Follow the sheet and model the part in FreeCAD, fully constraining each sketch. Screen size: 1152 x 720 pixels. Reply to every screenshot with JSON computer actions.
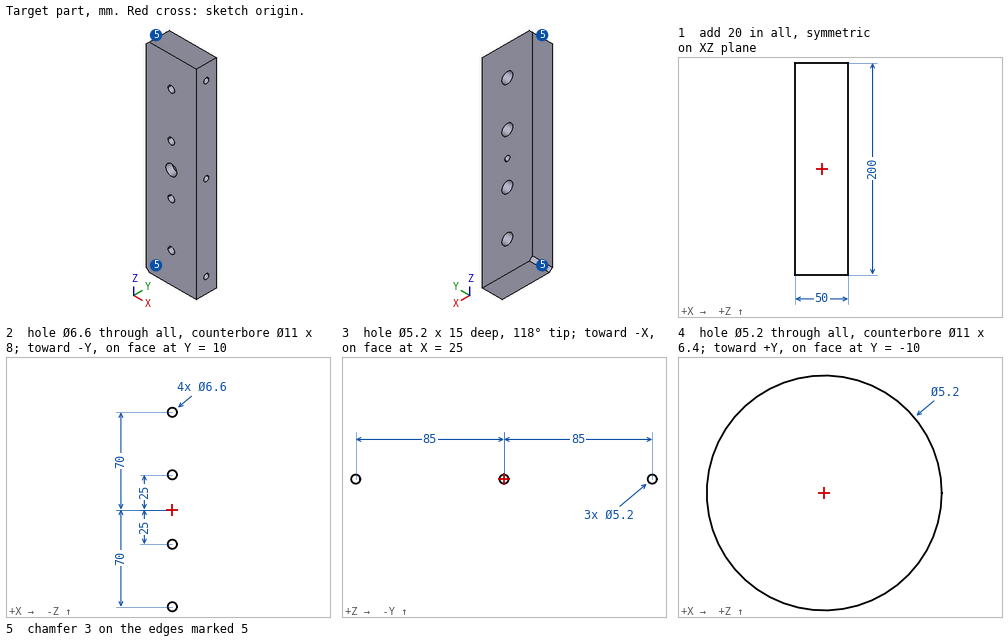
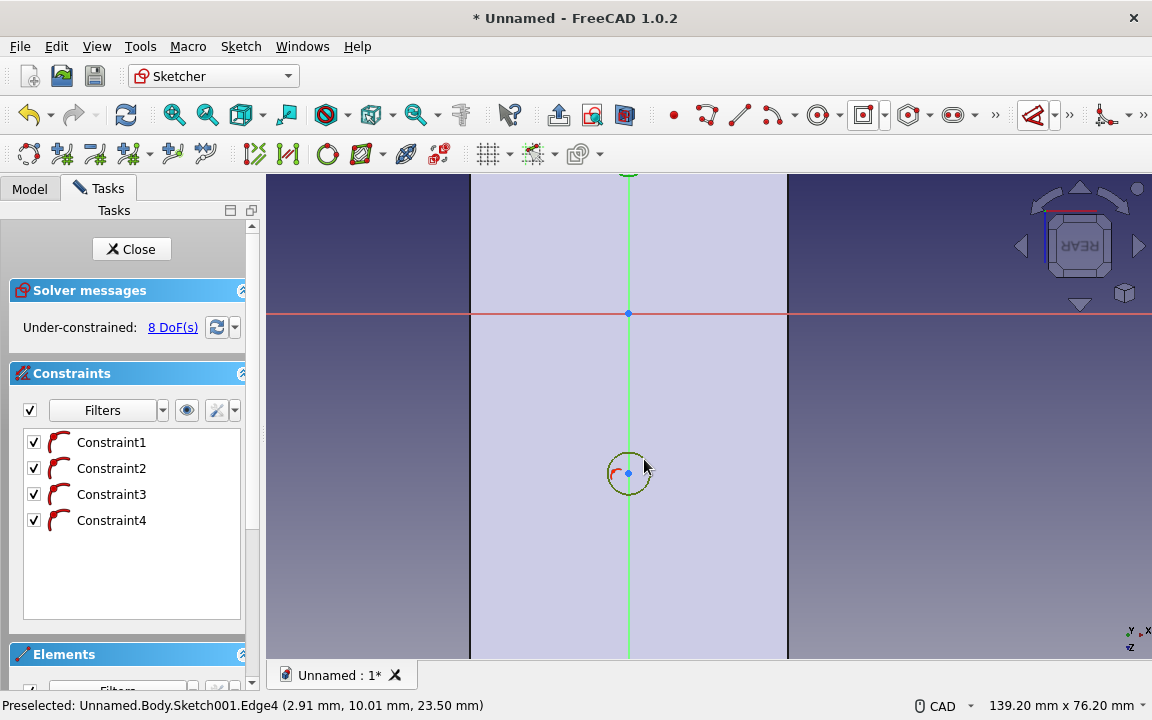
{"action": "key", "text": "e"}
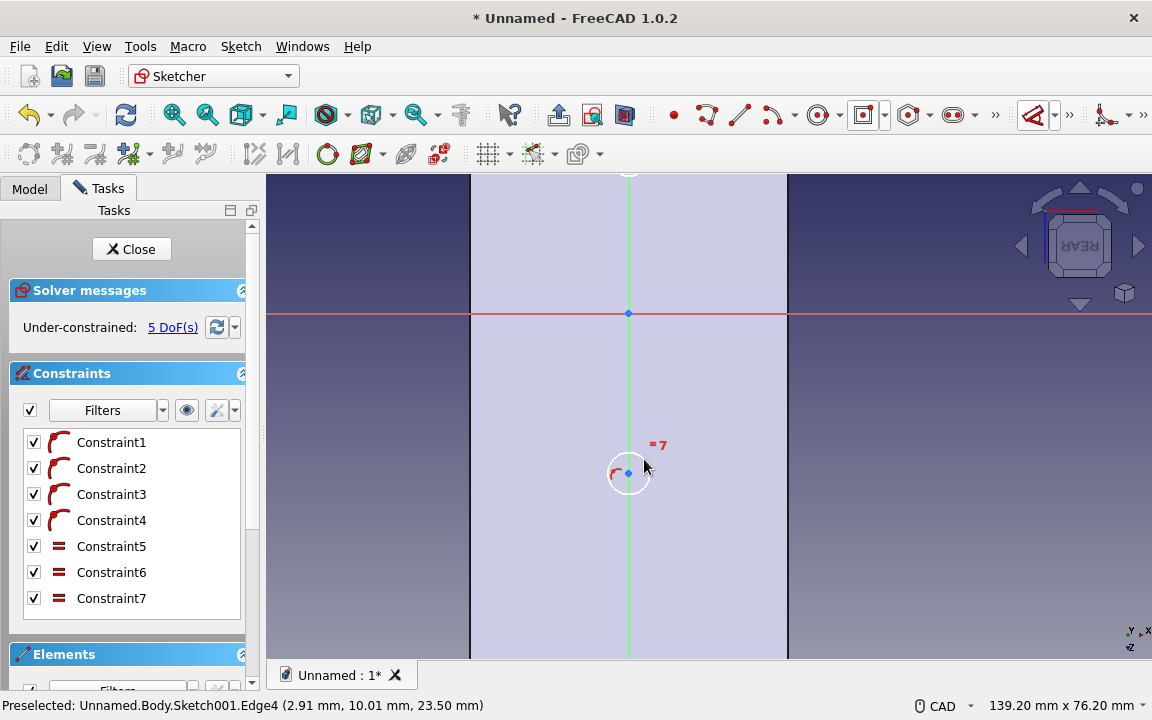
{"action": "scroll", "coordinate": [645, 461], "scroll_direction": "down", "scroll_amount": 6}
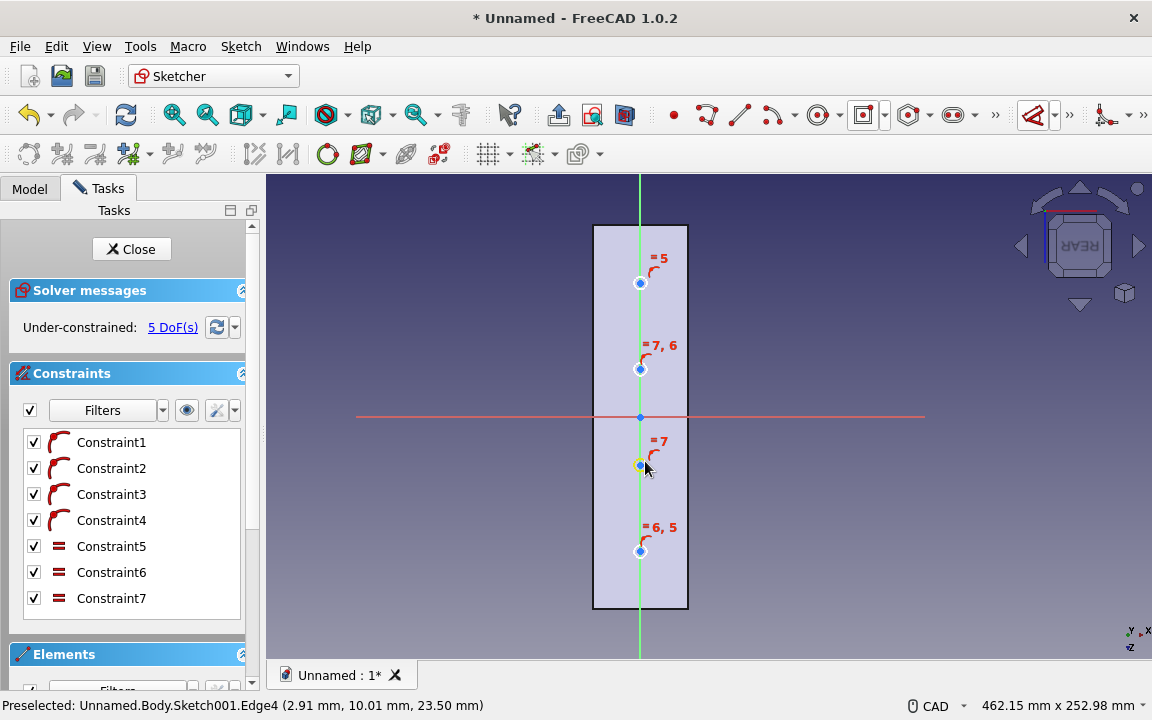
{"action": "scroll", "coordinate": [645, 279], "scroll_direction": "up", "scroll_amount": 6}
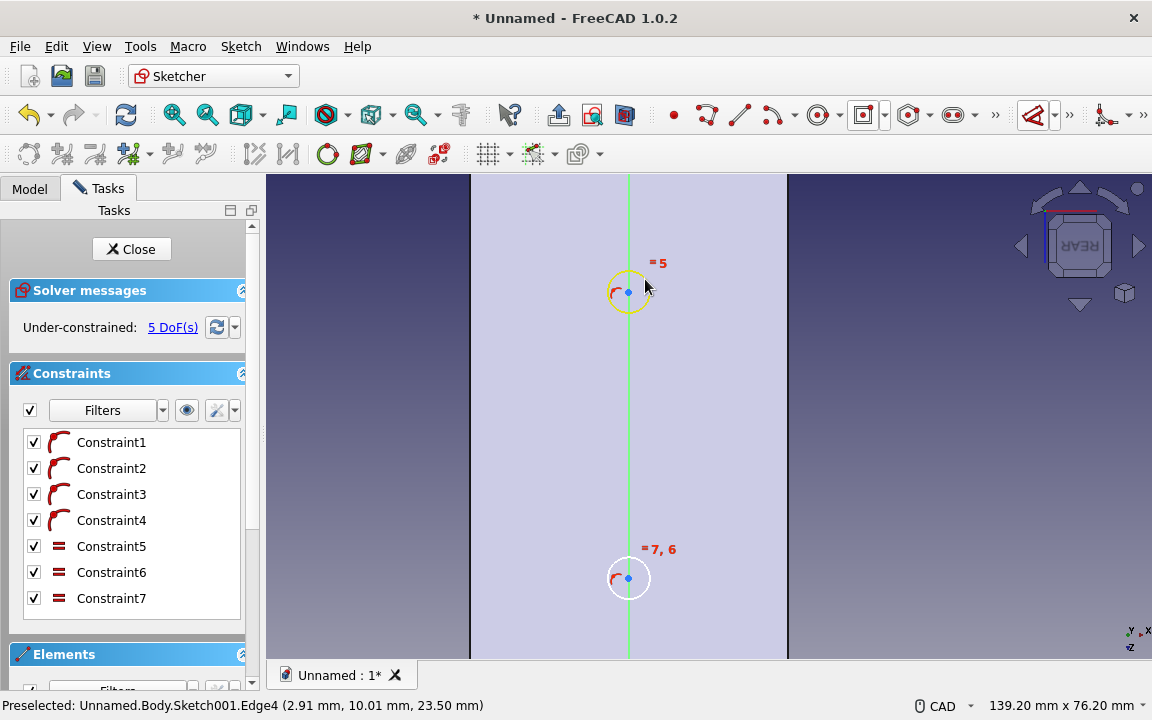
{"action": "left_click", "coordinate": [644, 277]}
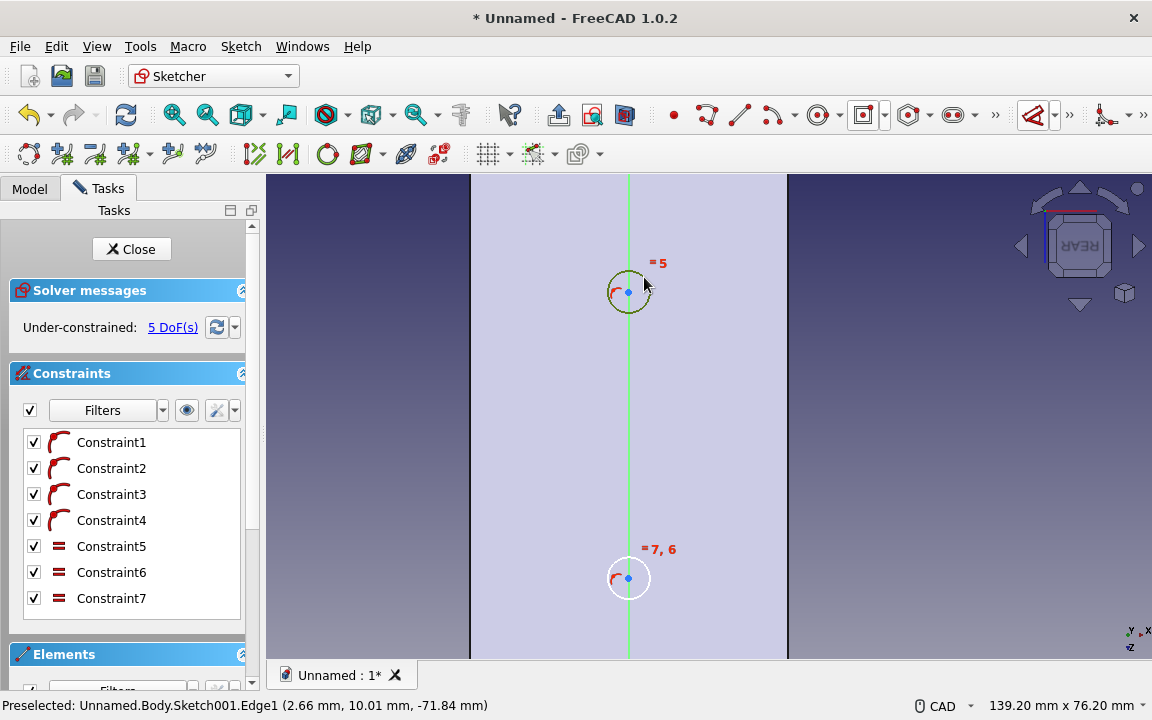
{"action": "left_click", "coordinate": [1054, 116]}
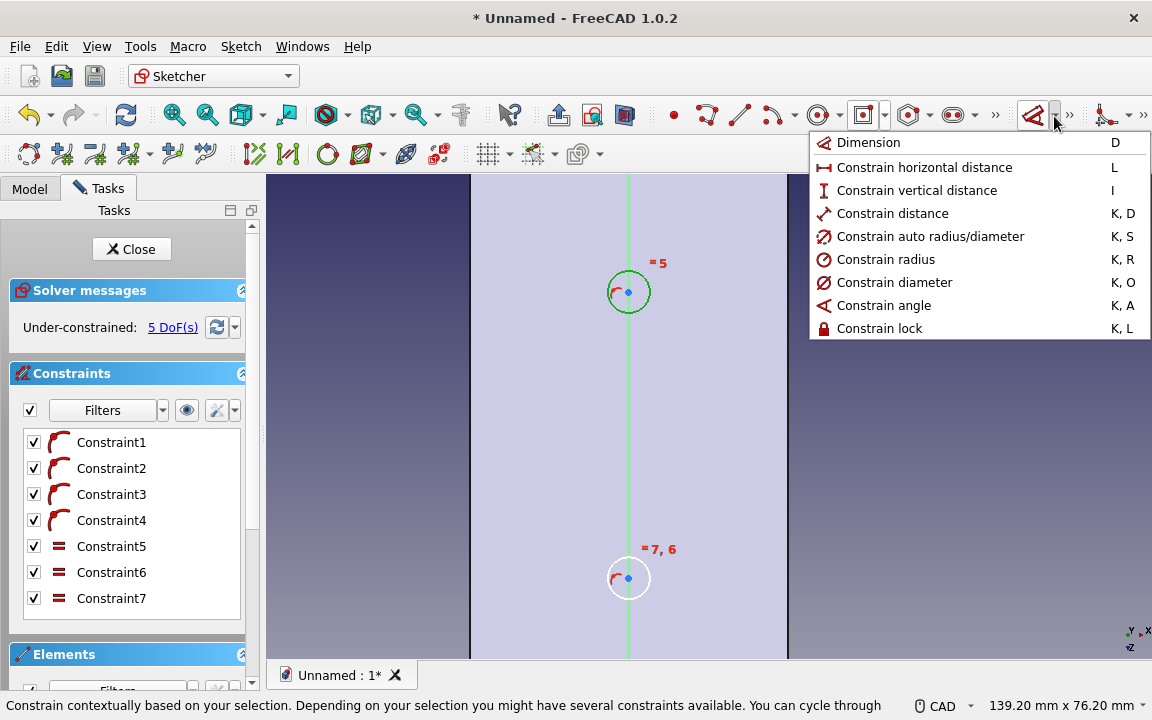
{"action": "left_click", "coordinate": [980, 282]}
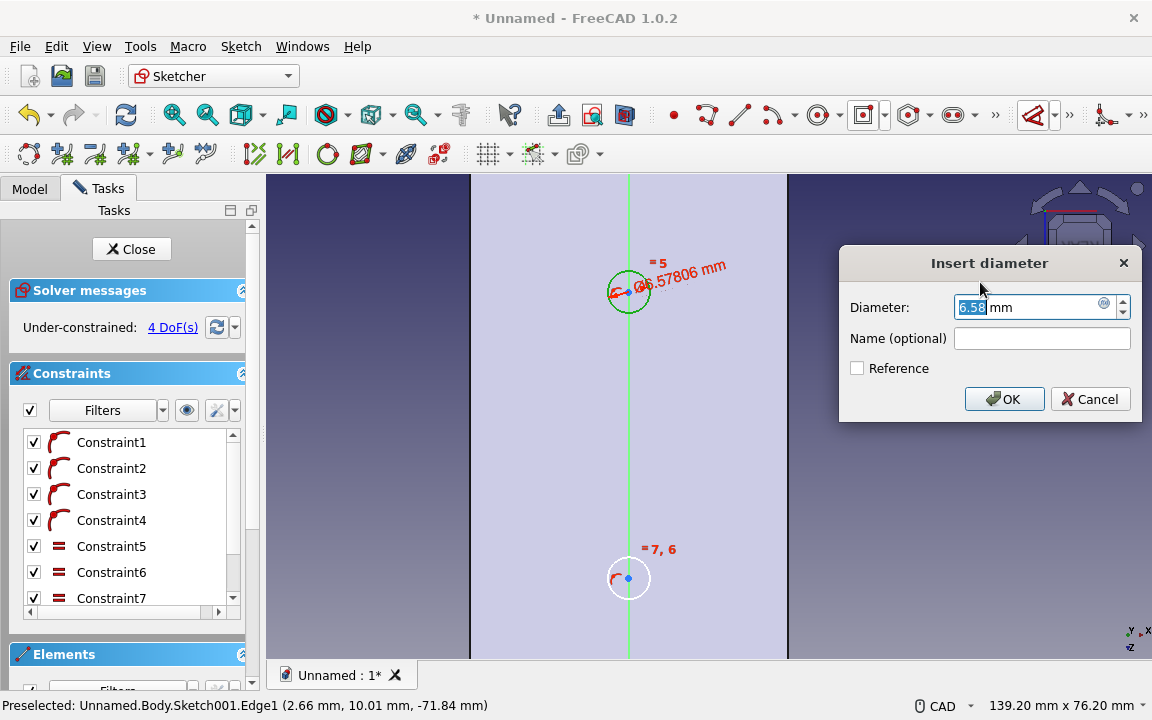
{"action": "type", "text": "6.6"}
{"action": "key", "text": "Return"}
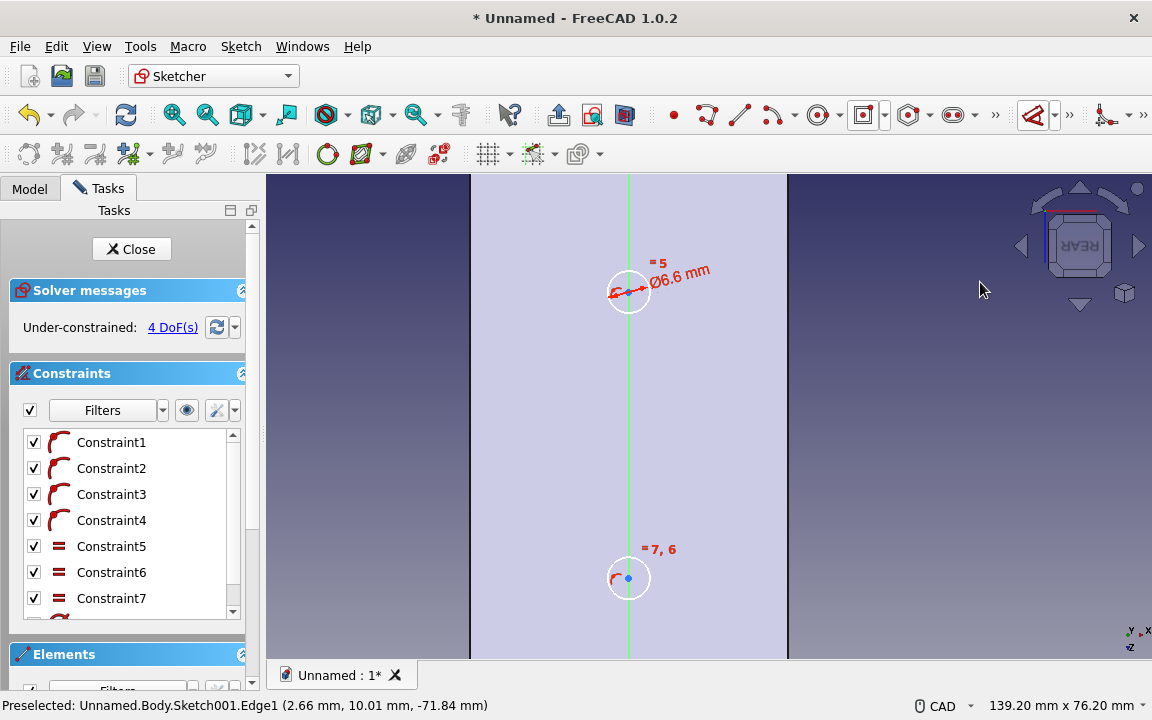
{"action": "left_click", "coordinate": [629, 292]}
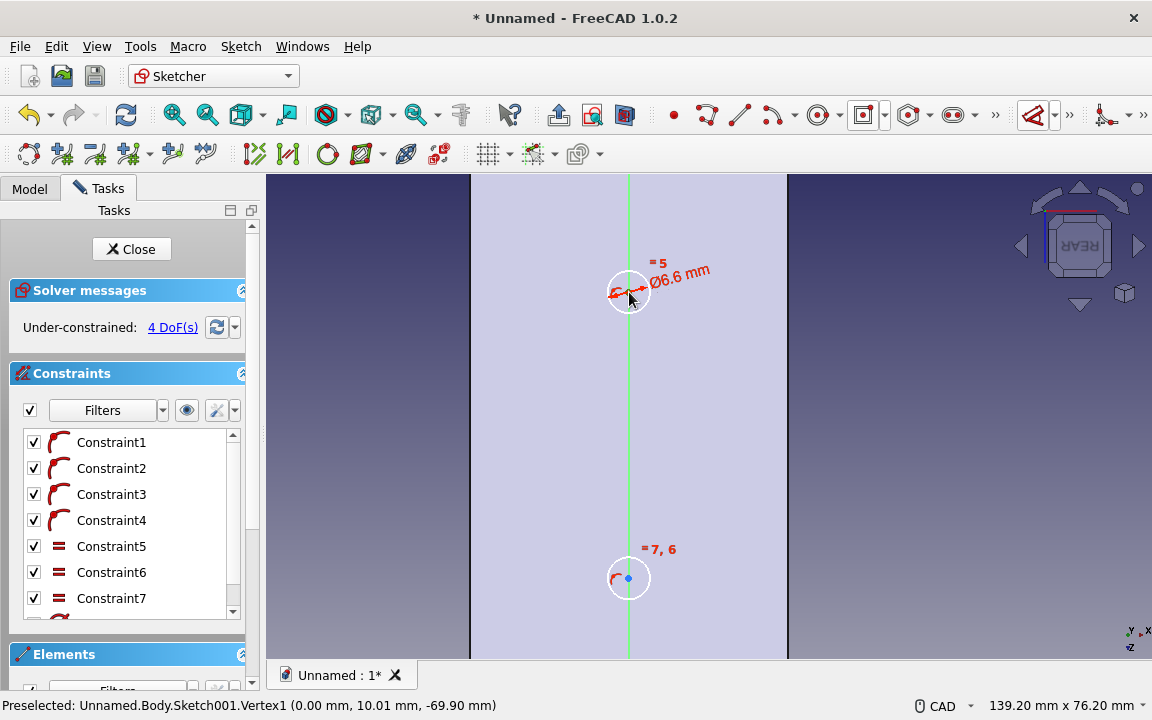
{"action": "key", "text": "i"}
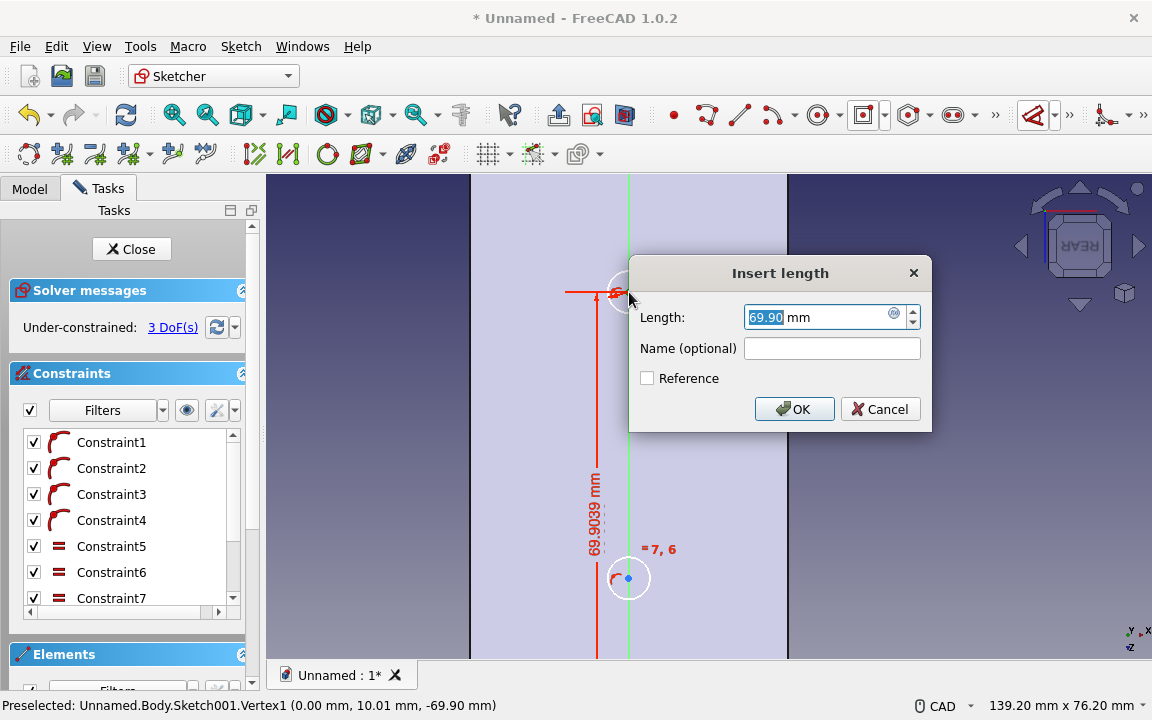
{"action": "type", "text": "70"}
{"action": "key", "text": "Return"}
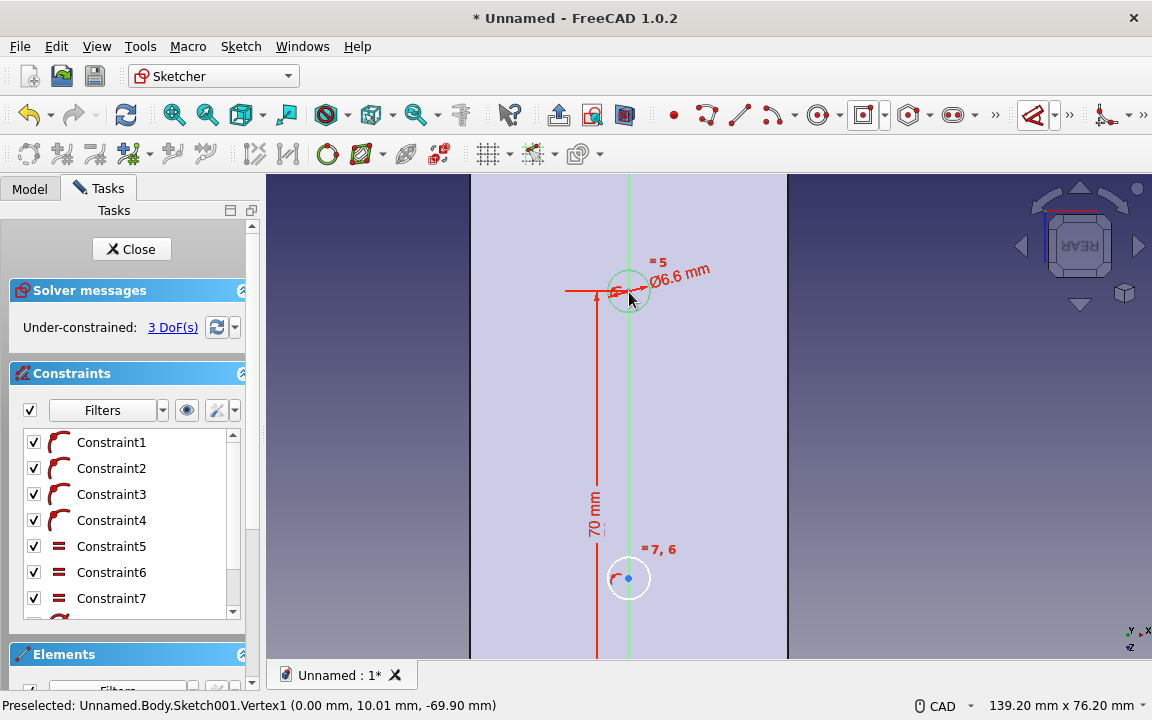
{"action": "scroll", "coordinate": [645, 278], "scroll_direction": "down", "scroll_amount": 6}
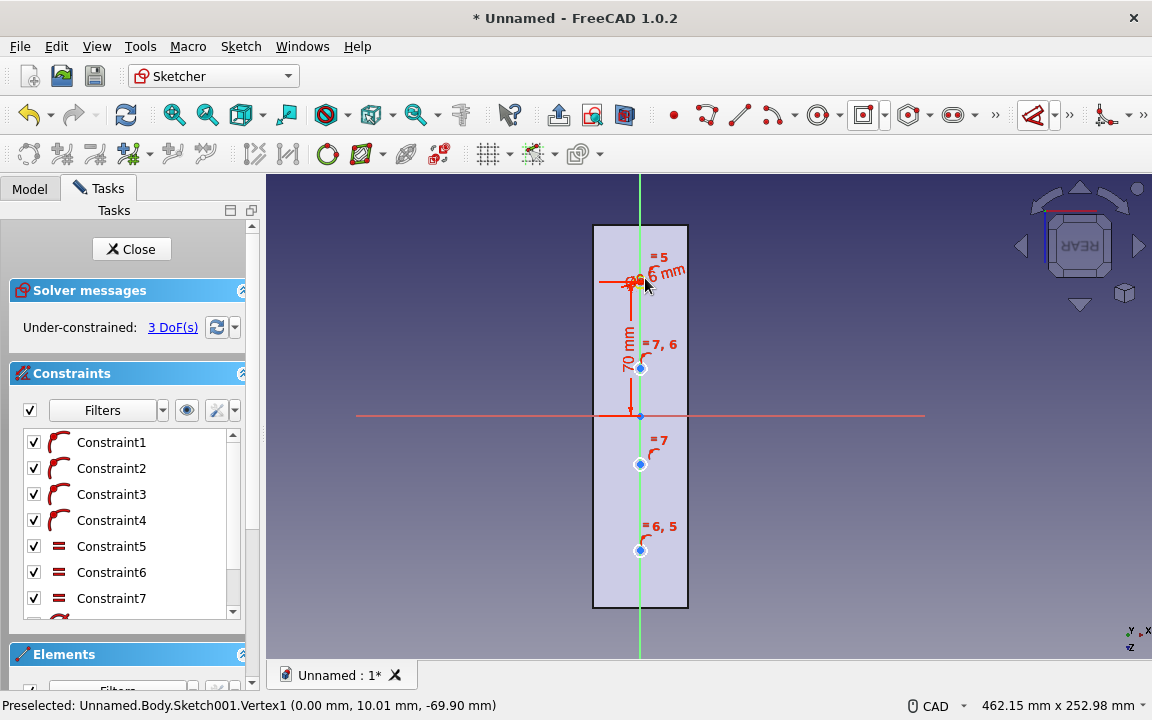
{"action": "left_click", "coordinate": [640, 551]}